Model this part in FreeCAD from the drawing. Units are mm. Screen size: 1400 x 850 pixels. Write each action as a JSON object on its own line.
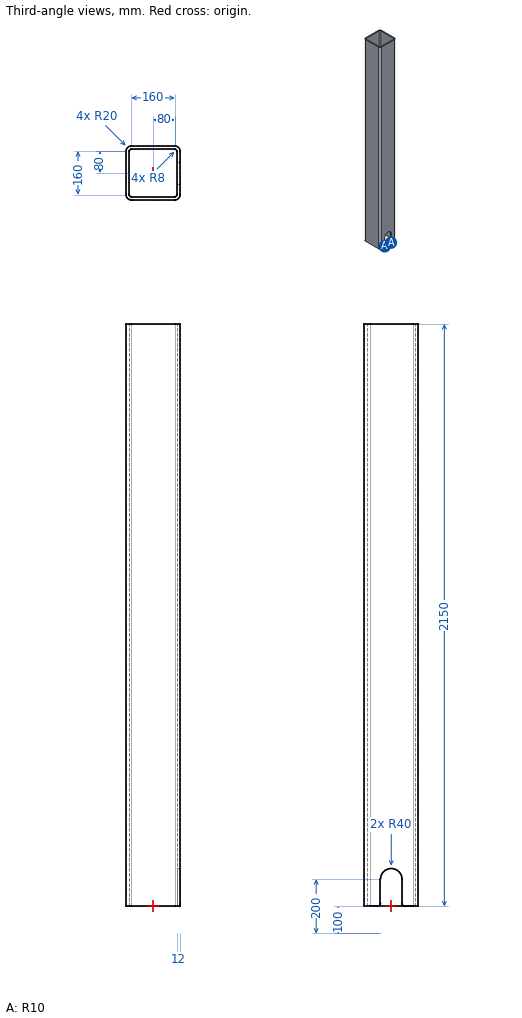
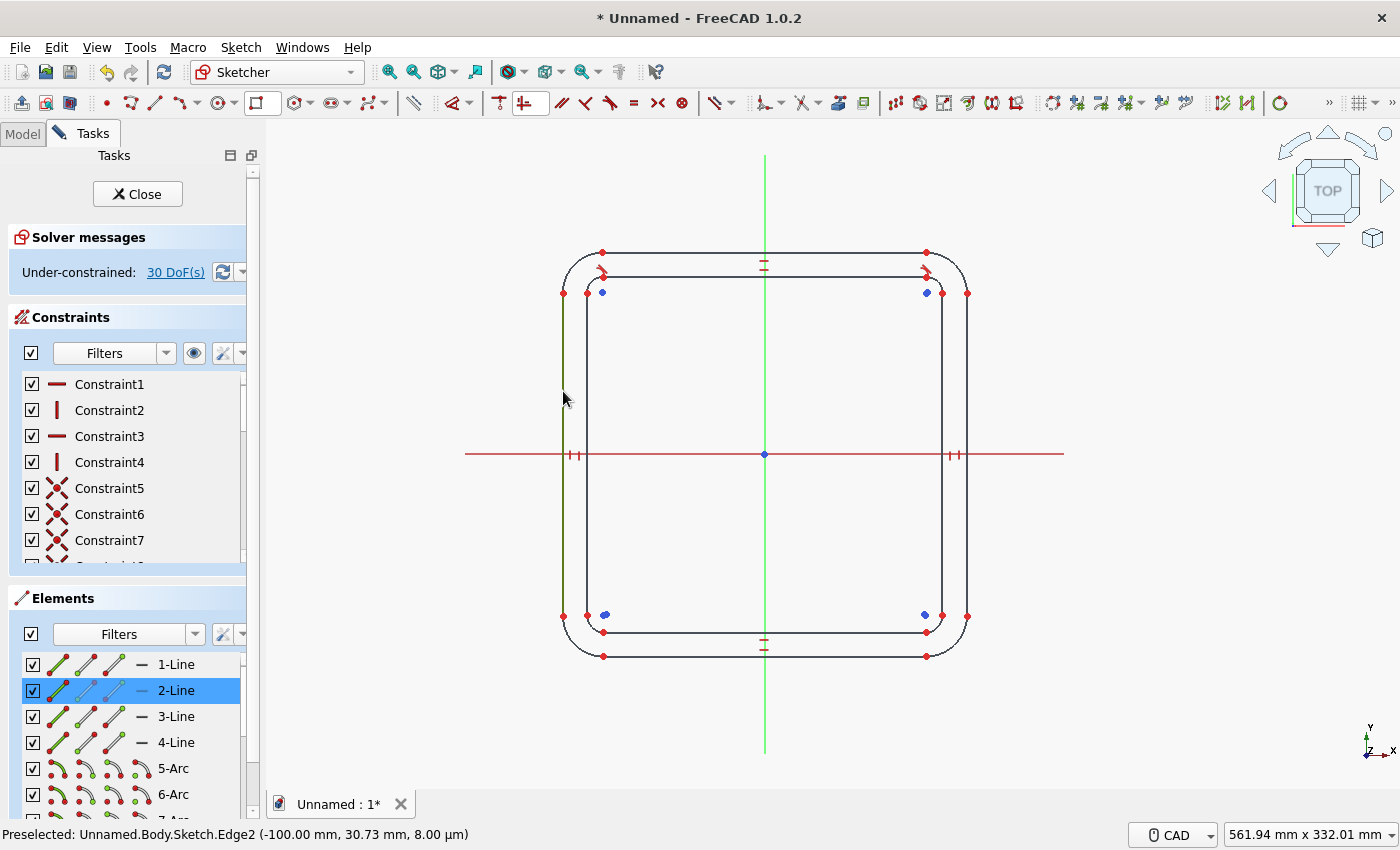
{"action": "left_click", "coordinate": [585, 257]}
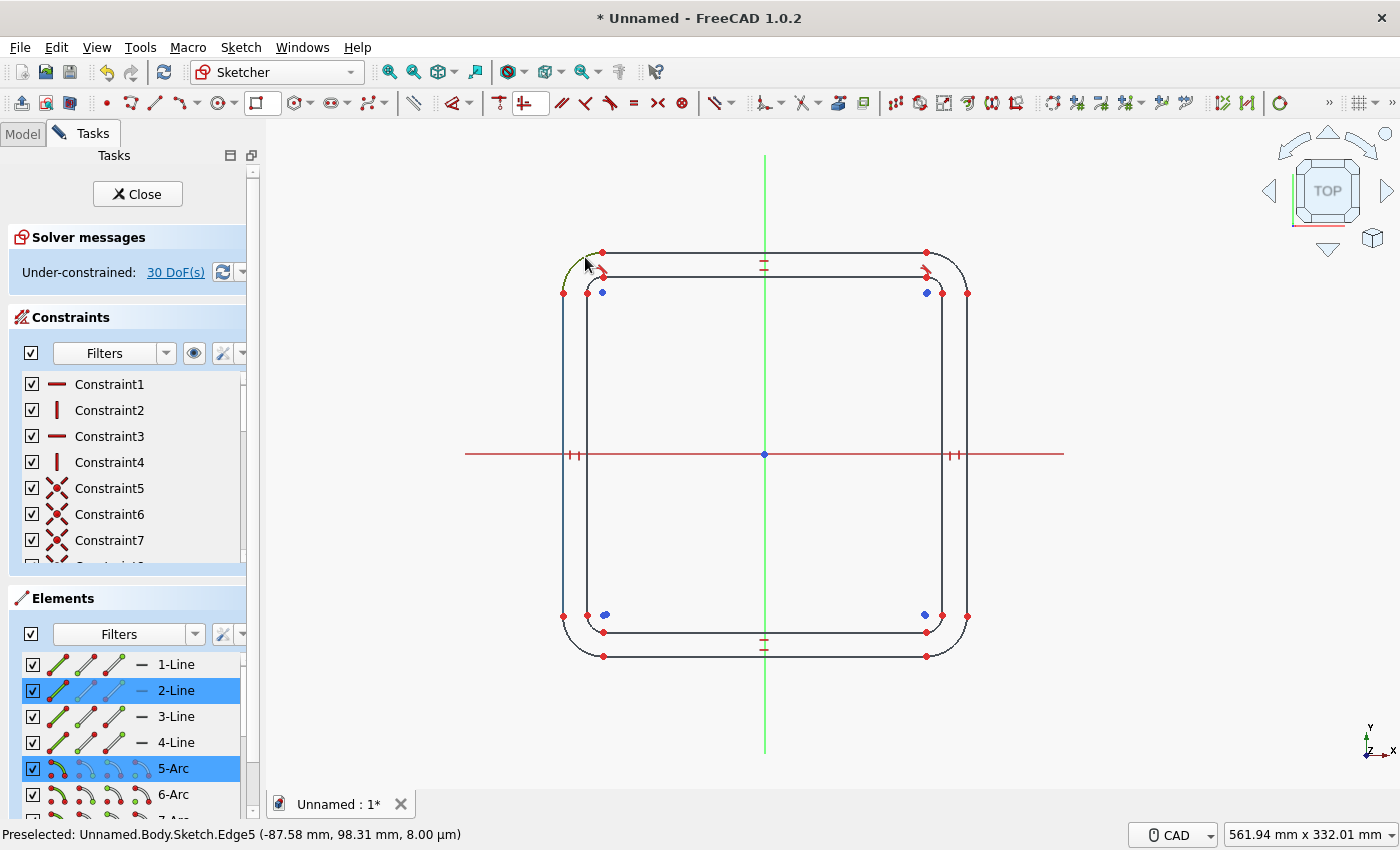
{"action": "left_click", "coordinate": [610, 104]}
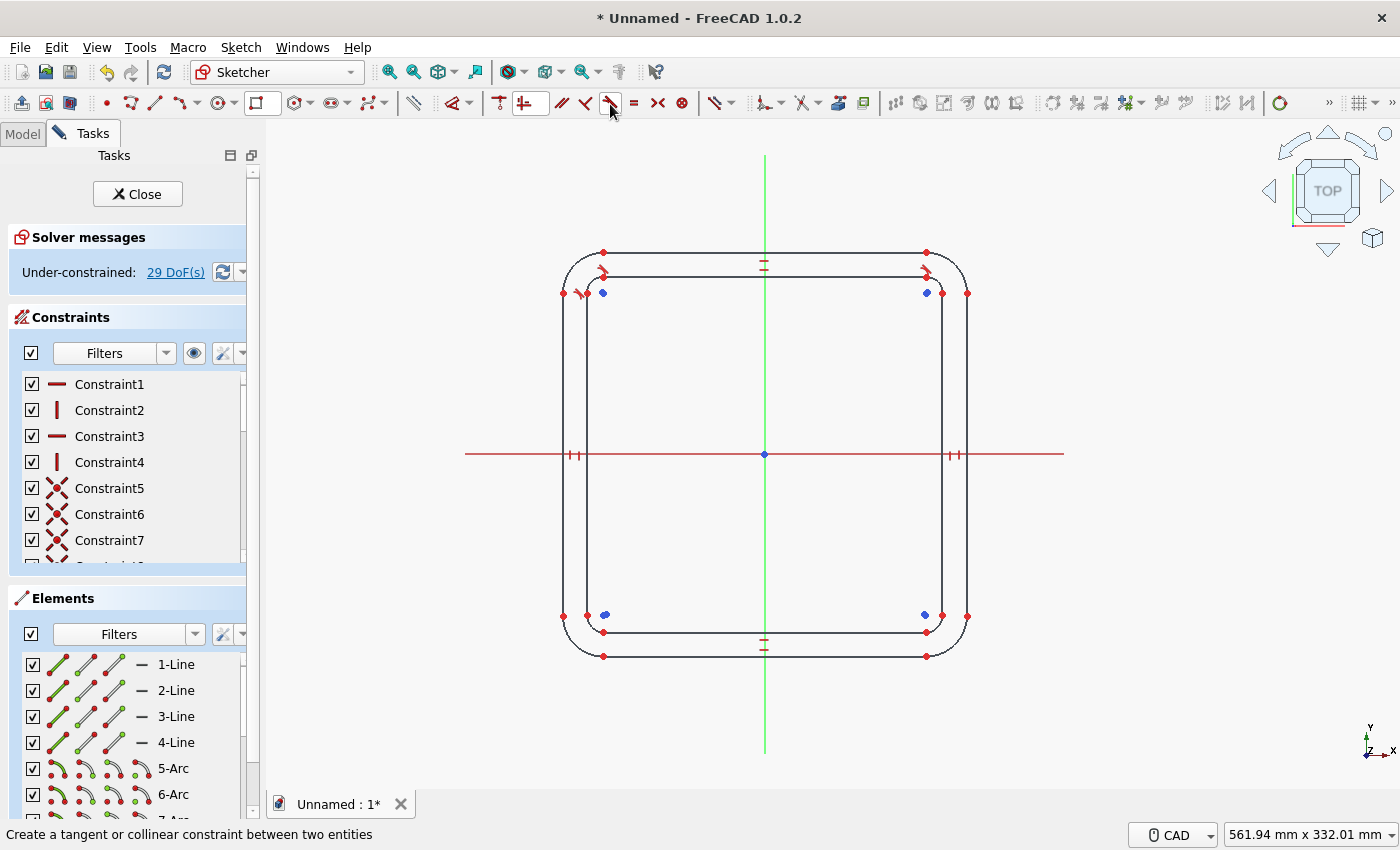
{"action": "left_click", "coordinate": [563, 391]}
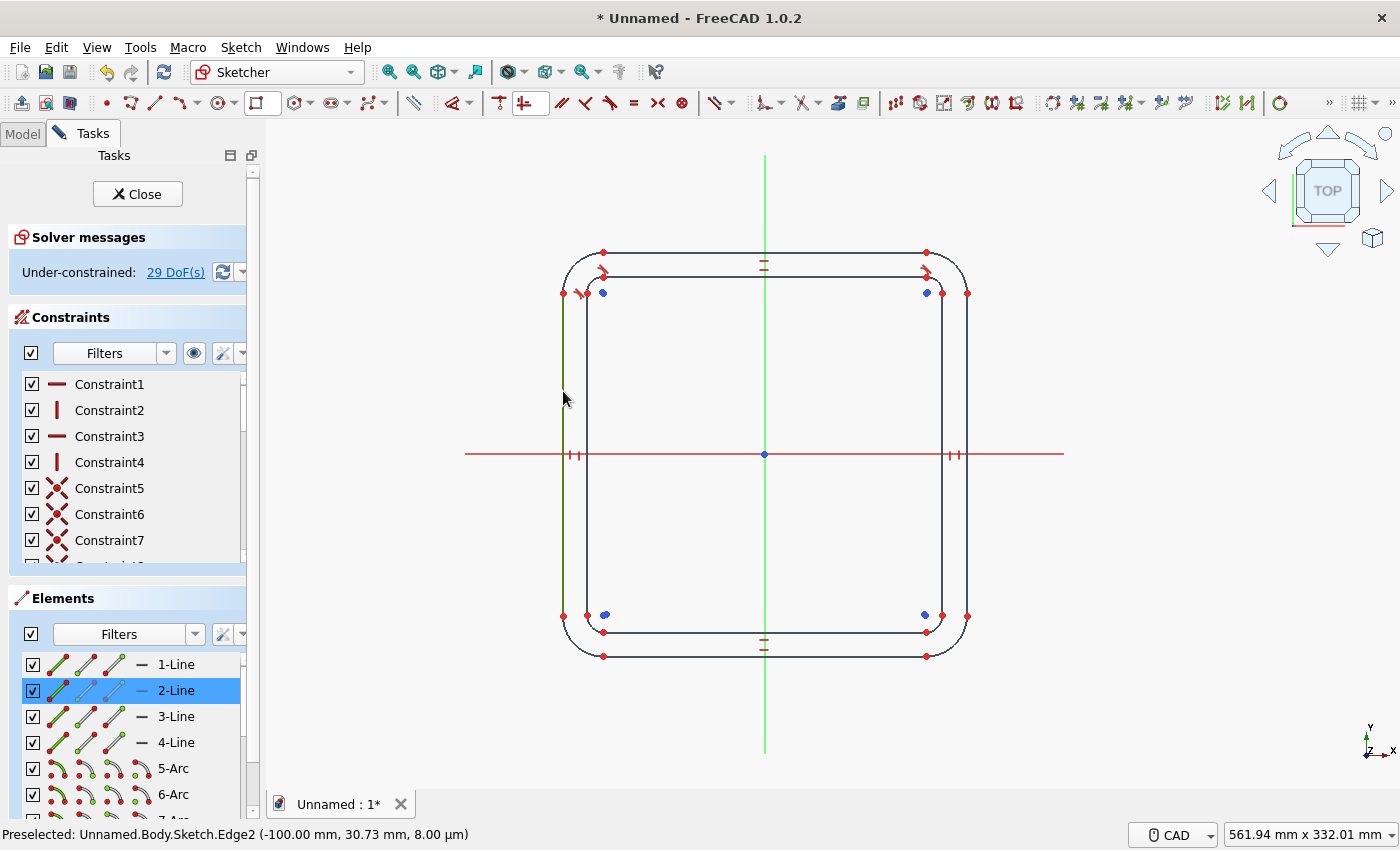
{"action": "left_click", "coordinate": [568, 635]}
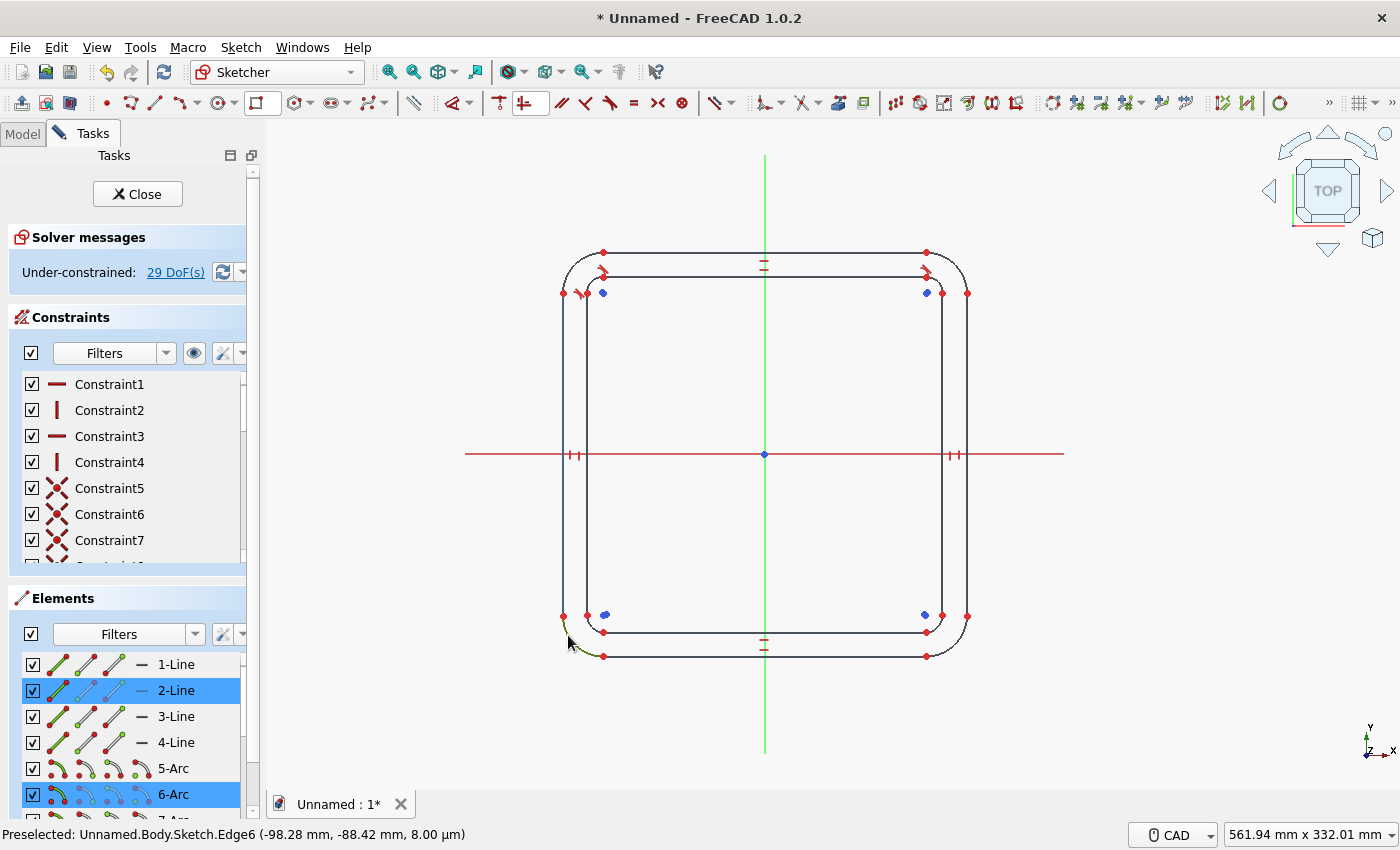
{"action": "left_click", "coordinate": [610, 104]}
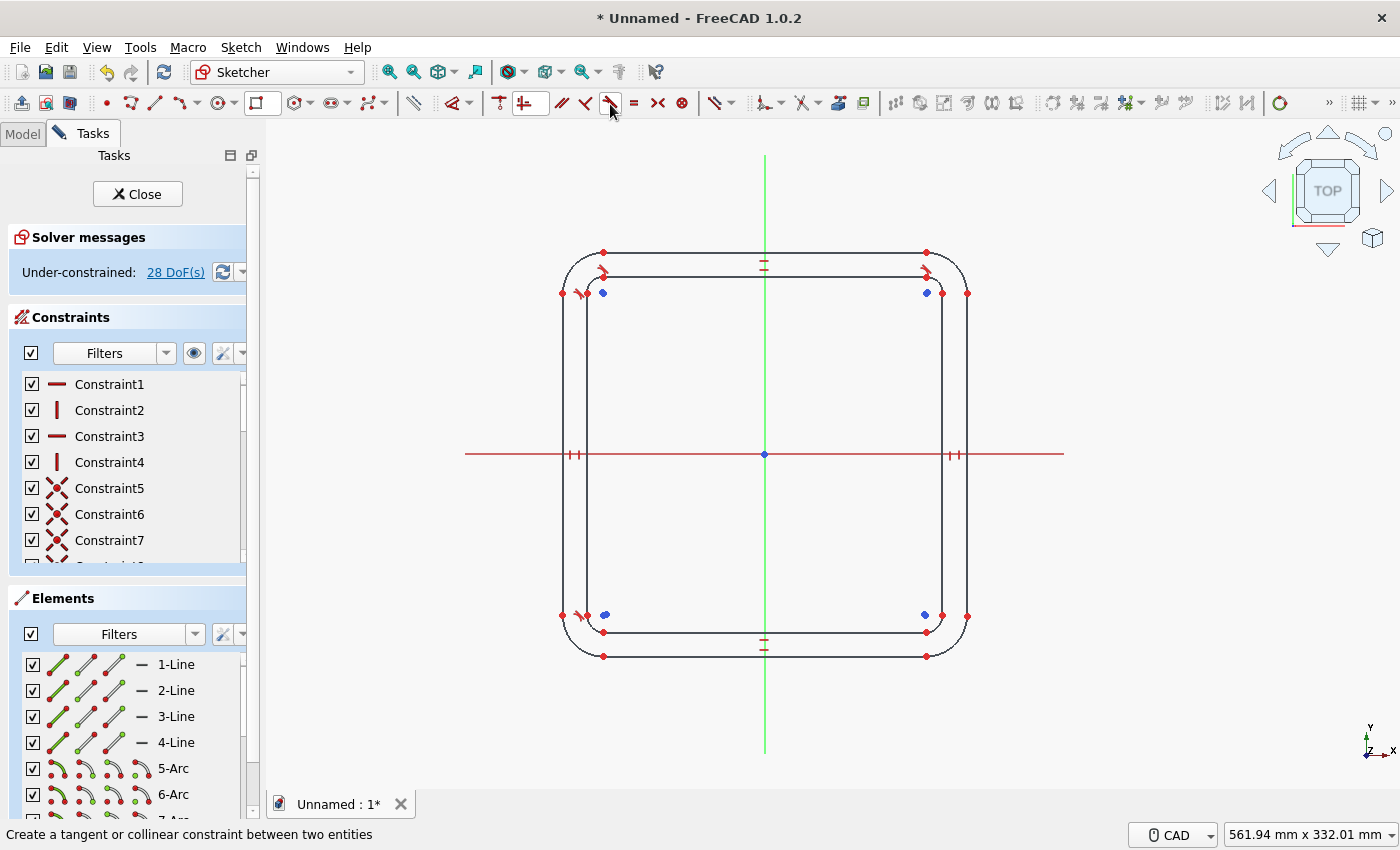
{"action": "left_click", "coordinate": [700, 657]}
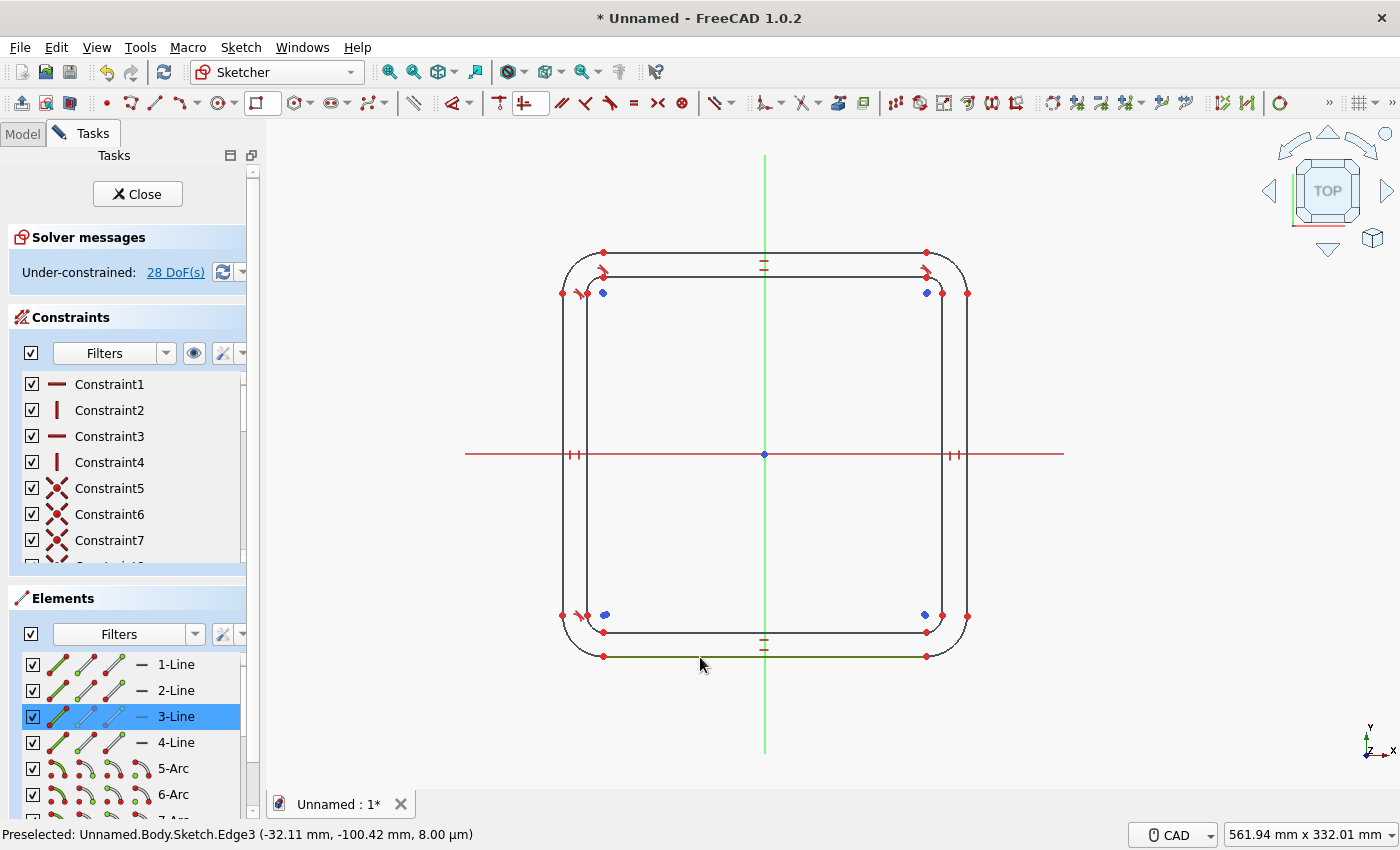
{"action": "left_click", "coordinate": [567, 634]}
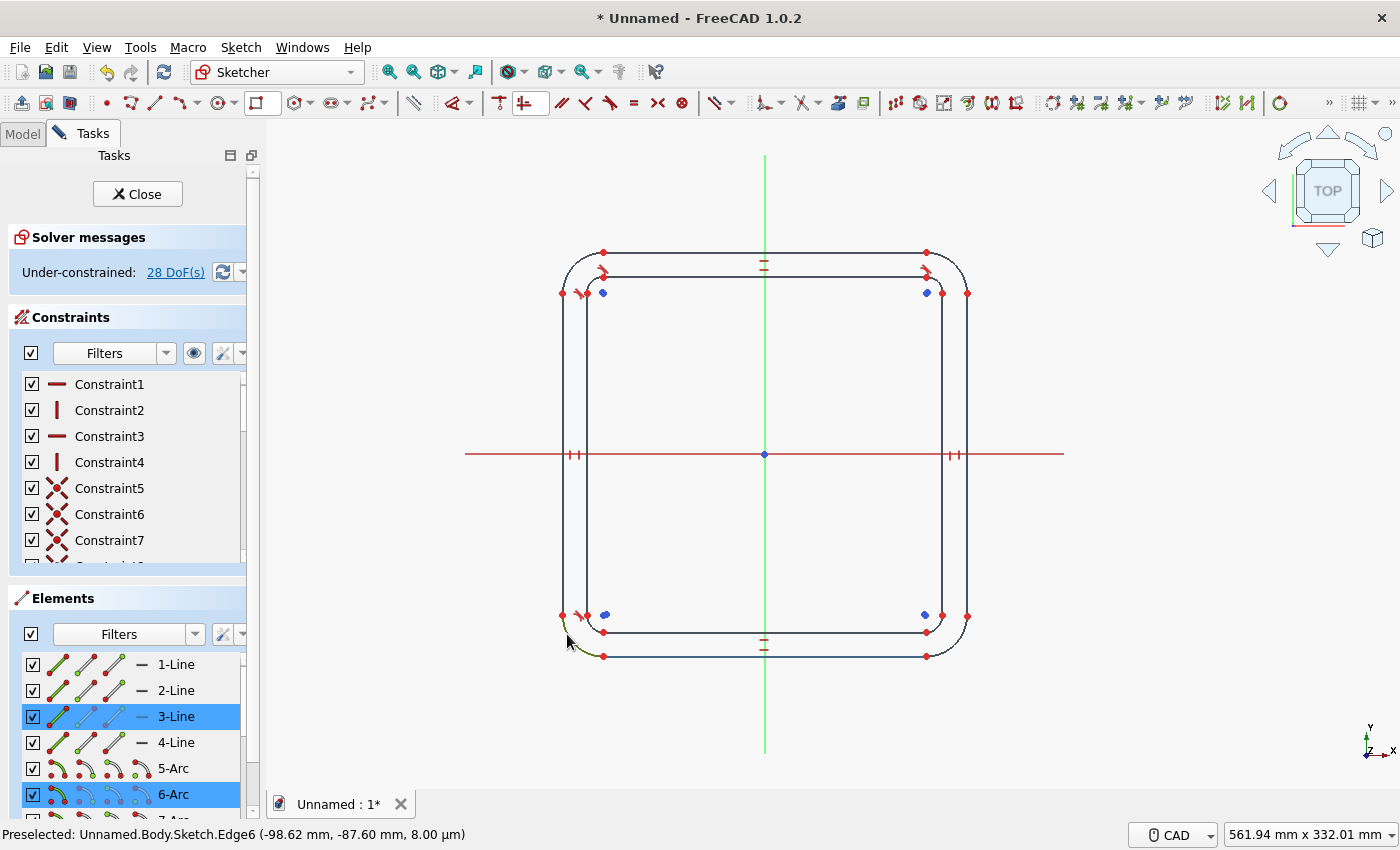
{"action": "left_click", "coordinate": [610, 104]}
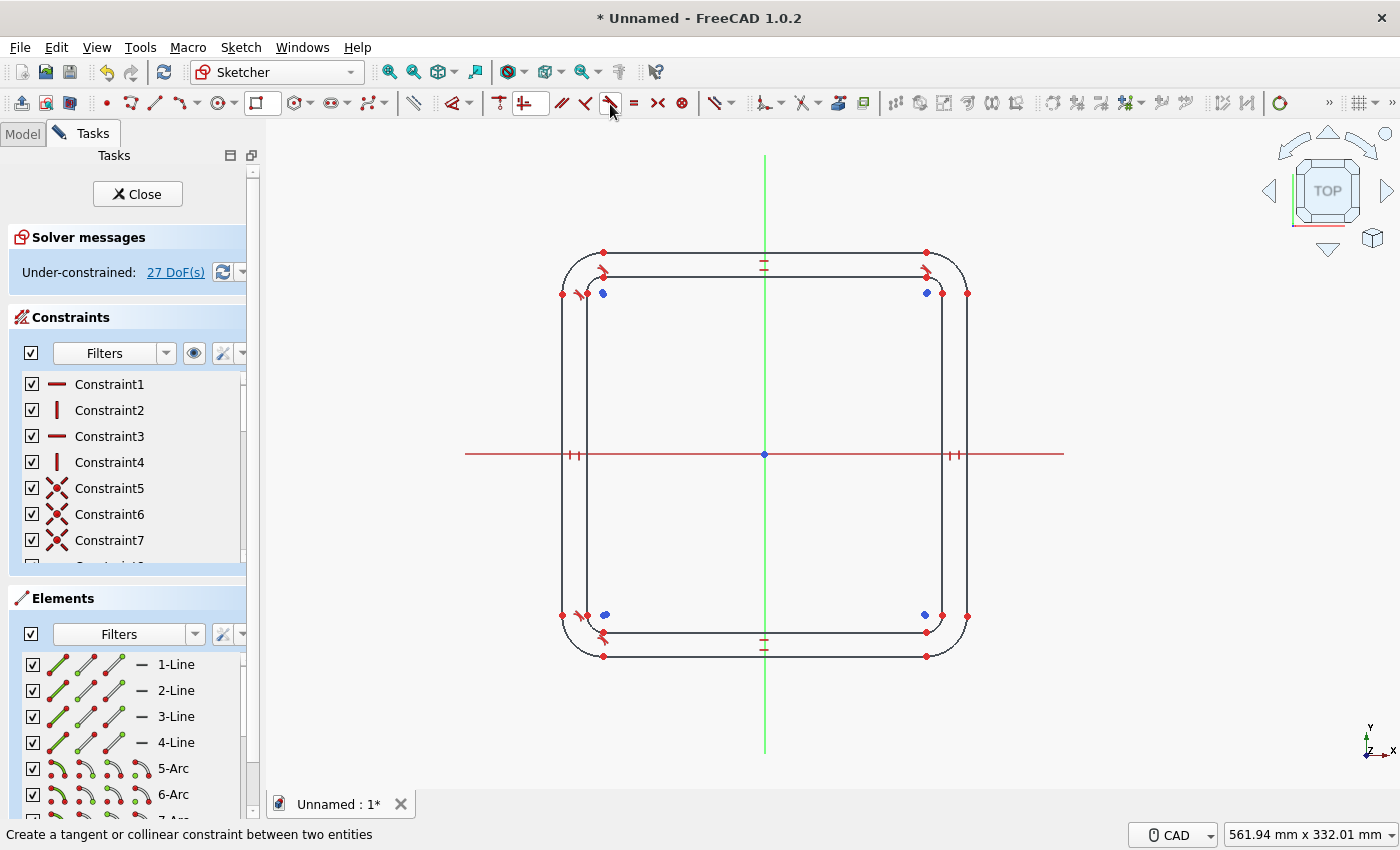
{"action": "left_click", "coordinate": [700, 657]}